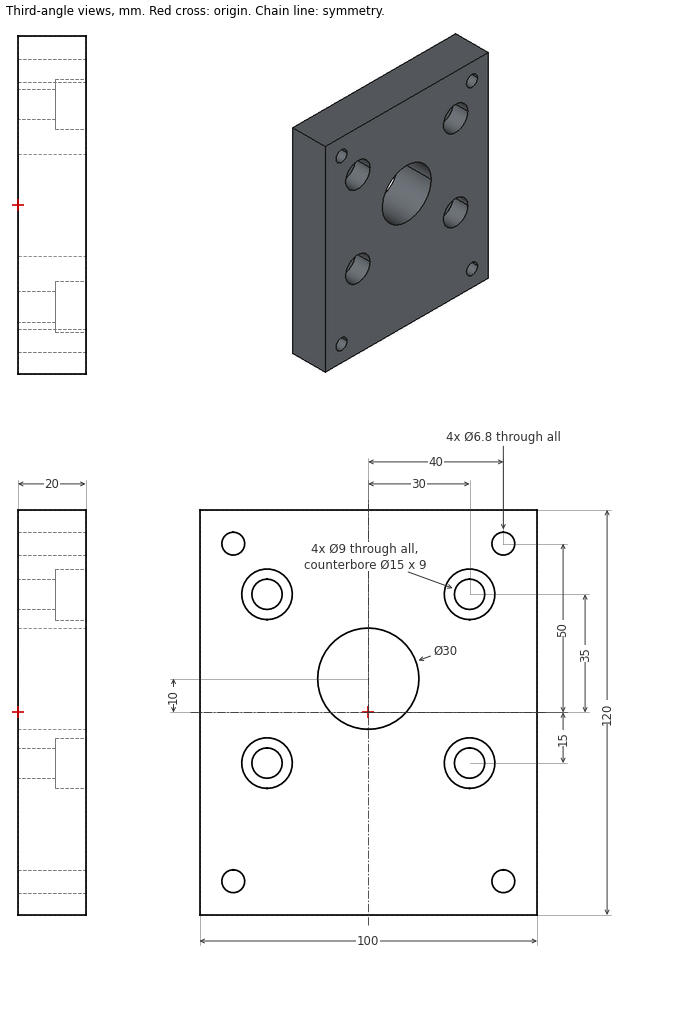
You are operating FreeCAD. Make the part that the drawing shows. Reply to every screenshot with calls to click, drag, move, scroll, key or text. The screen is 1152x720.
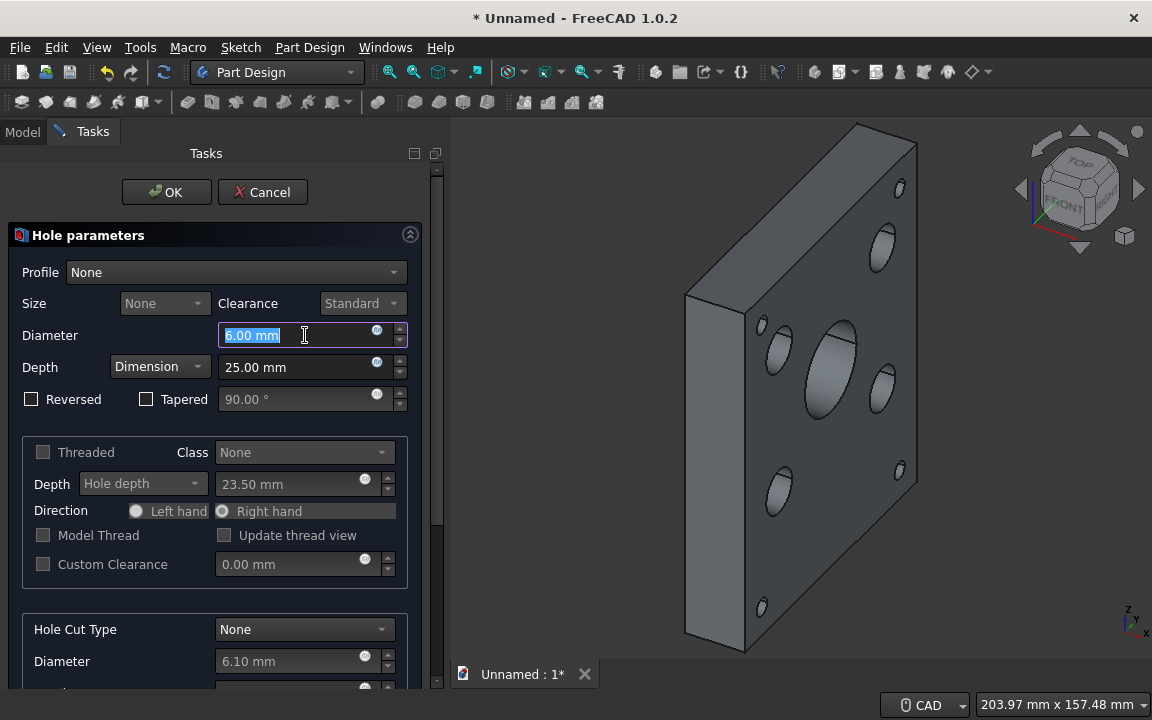
text(6.8)
key(Tab)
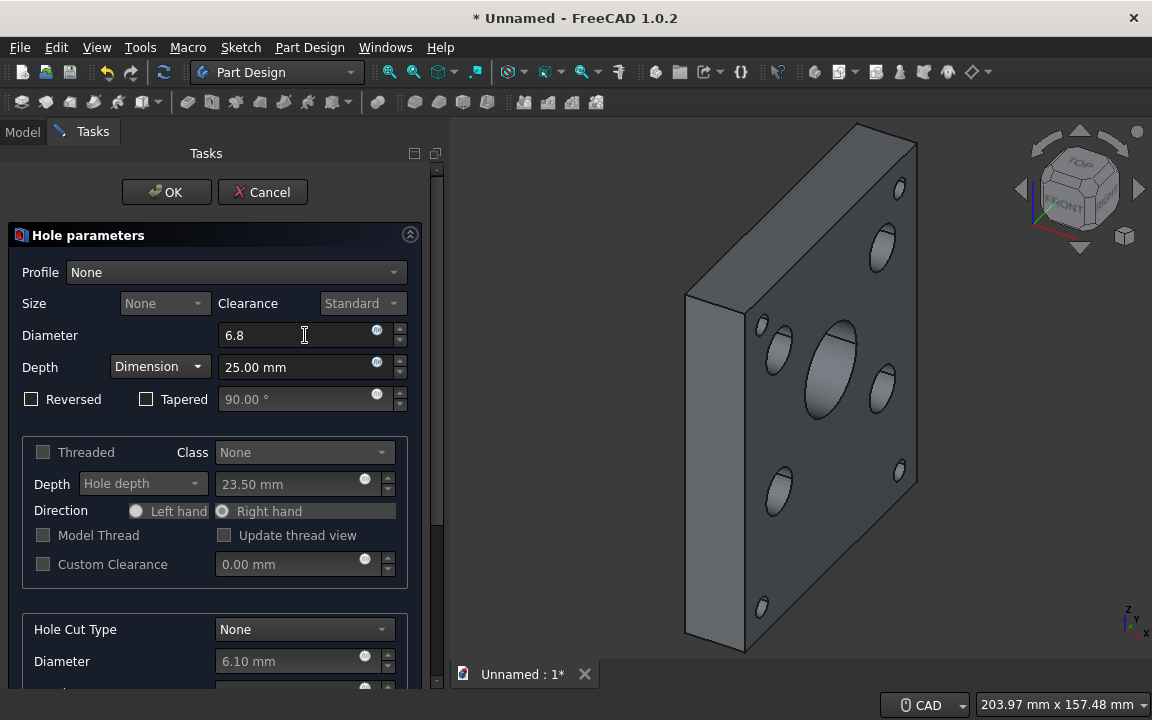
click(161, 366)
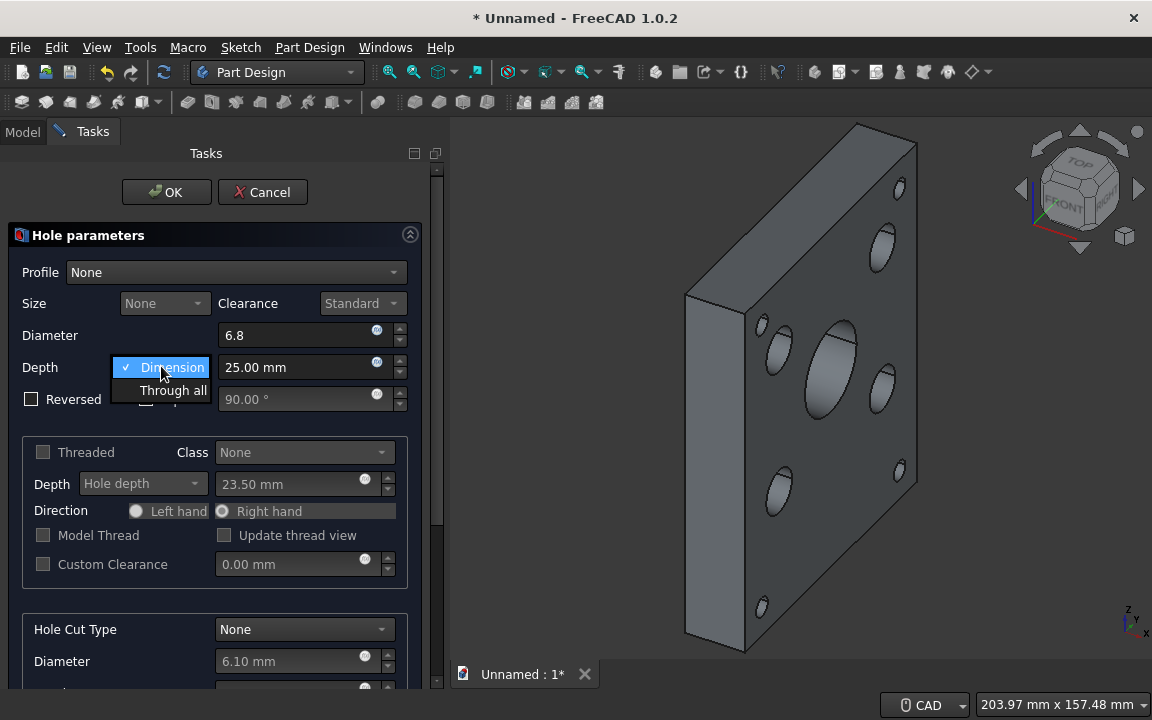
click(160, 390)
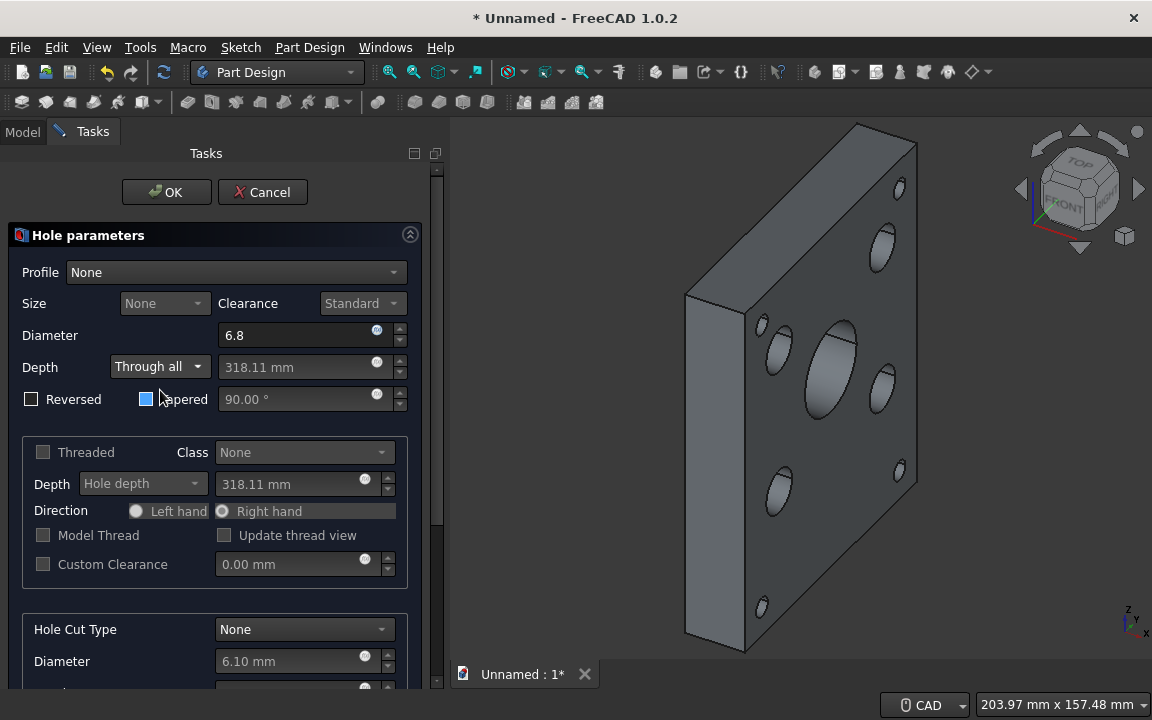
click(167, 192)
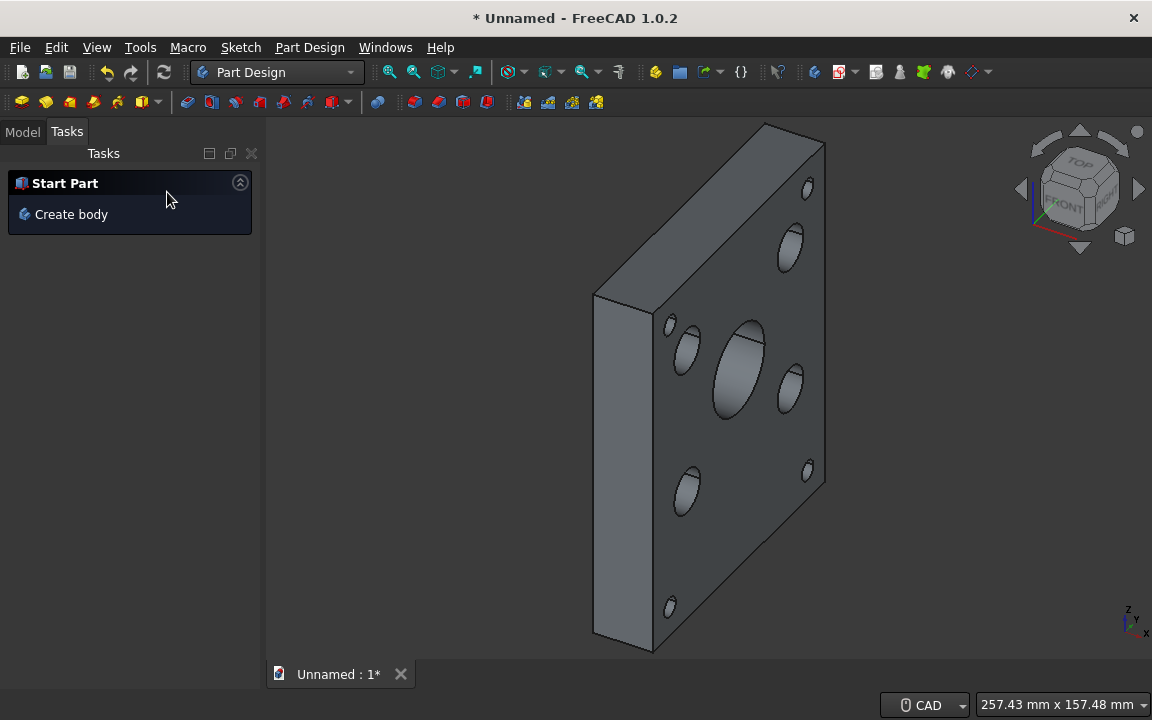
key(0)